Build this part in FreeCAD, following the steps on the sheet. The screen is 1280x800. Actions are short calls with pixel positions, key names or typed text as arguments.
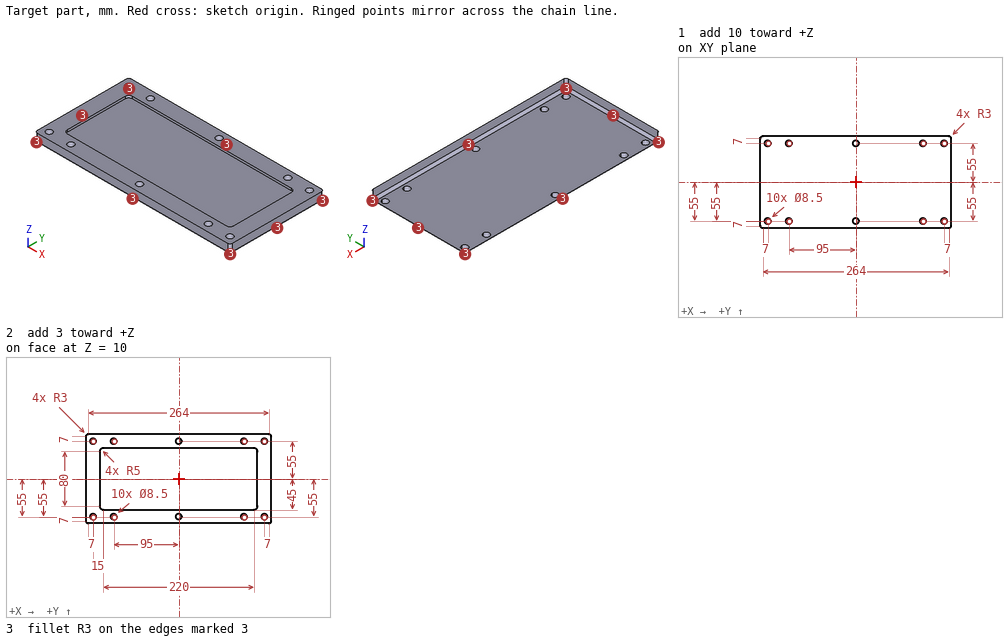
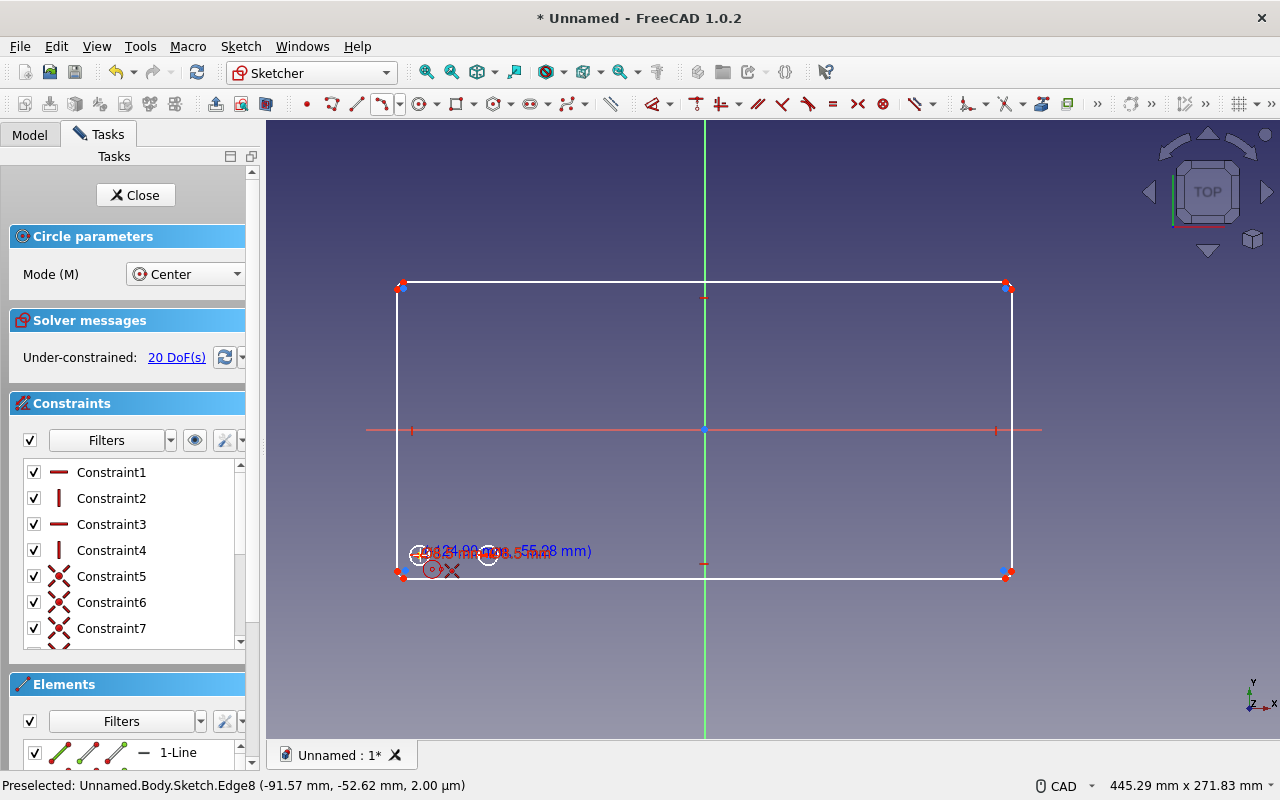
scroll(705, 555, up, 5)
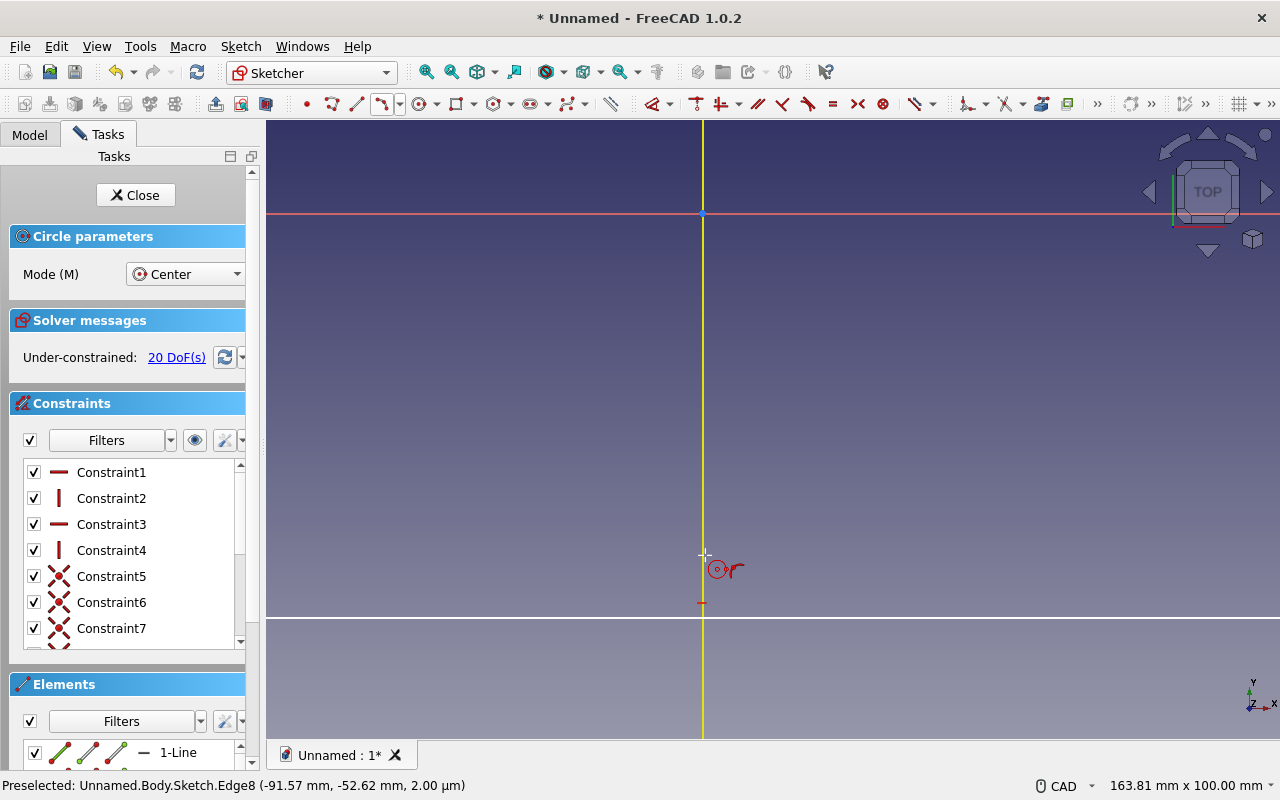
click(703, 554)
move(722, 536)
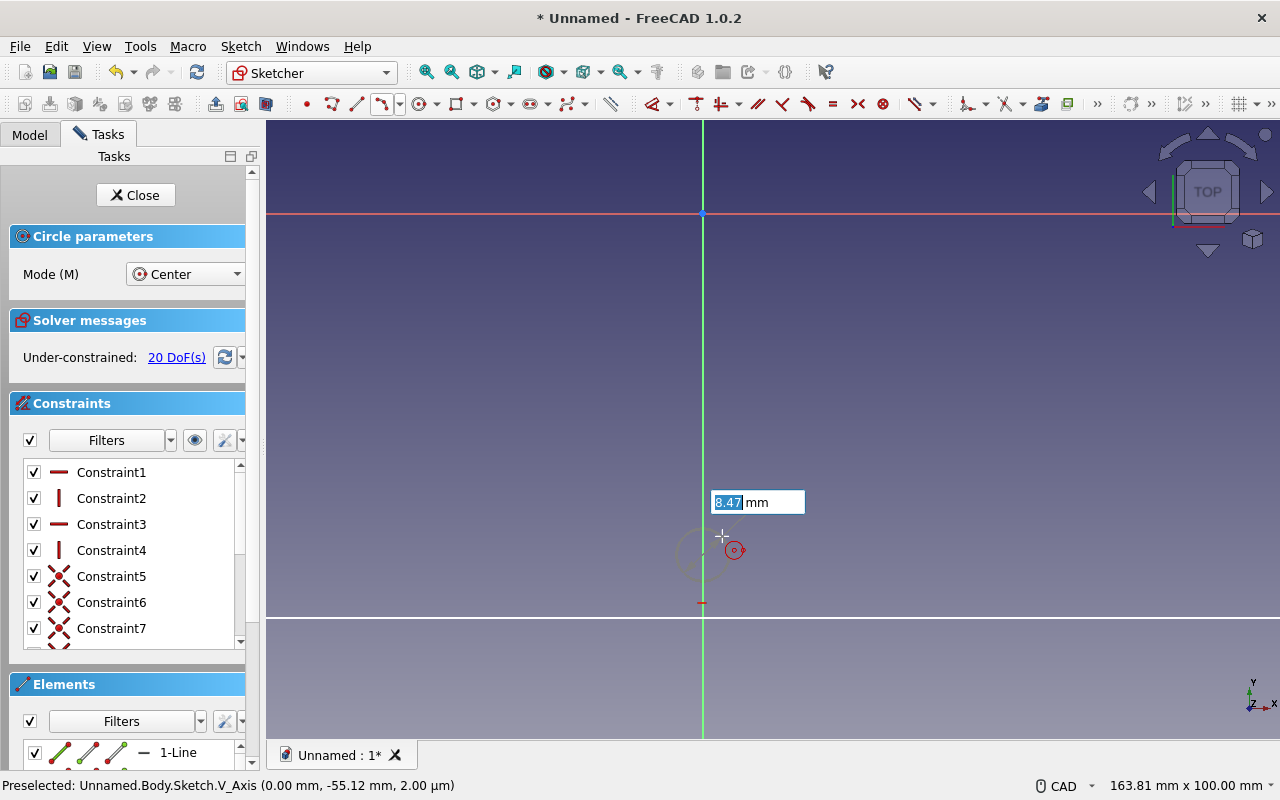
text(8.5)
key(Return)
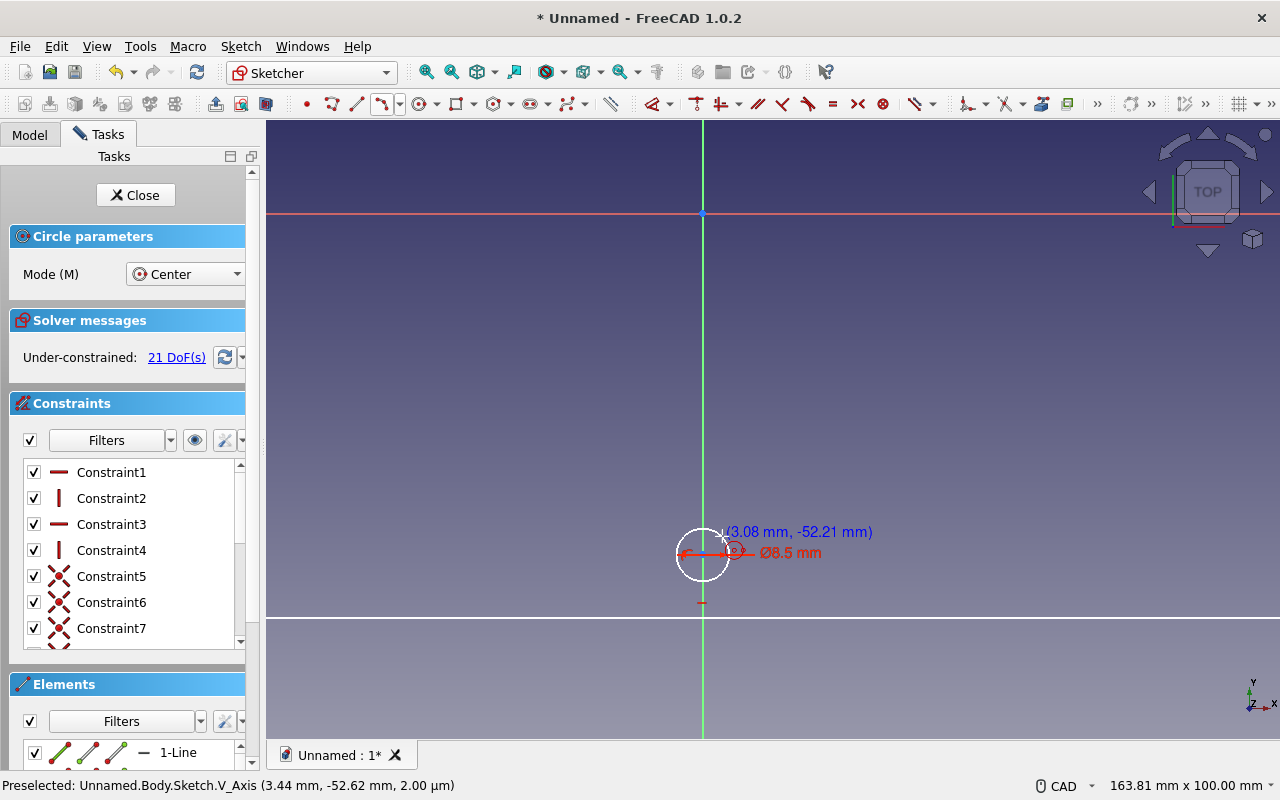
scroll(705, 555, down, 5)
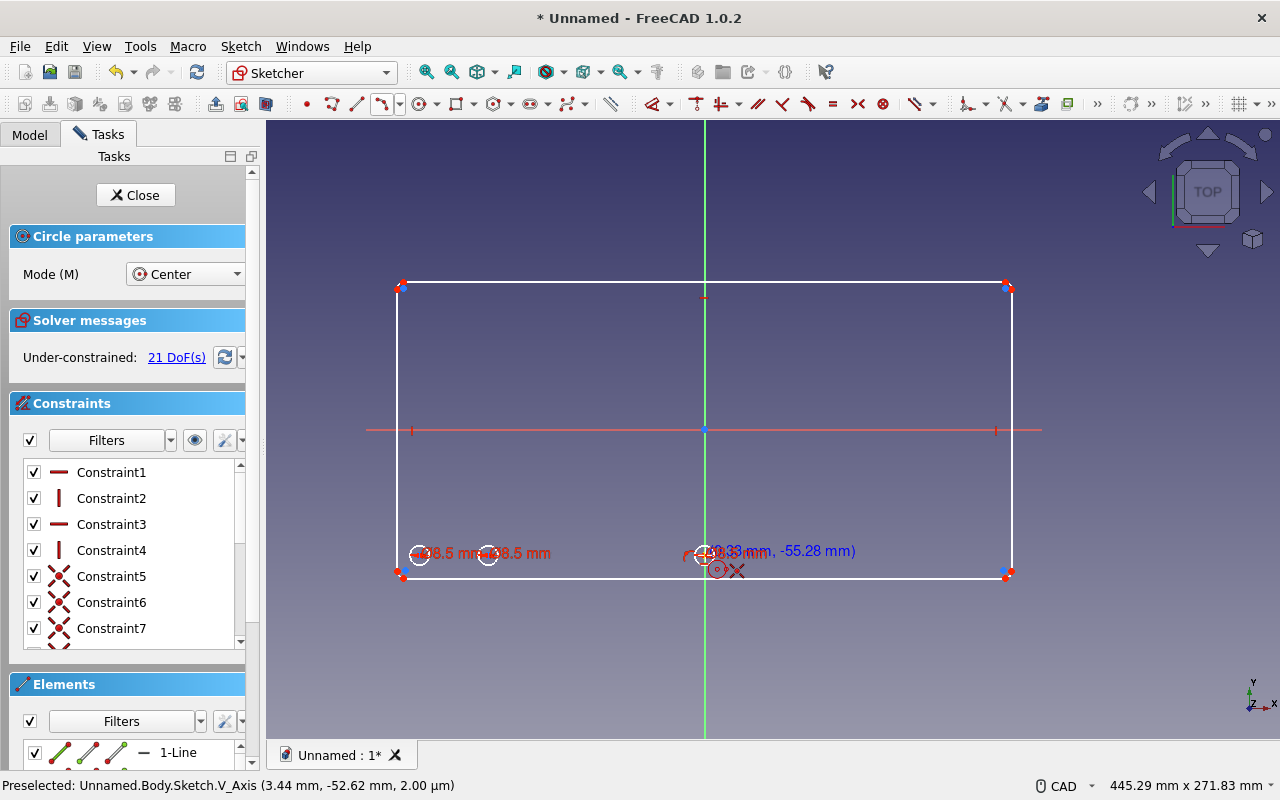
scroll(921, 555, up, 5)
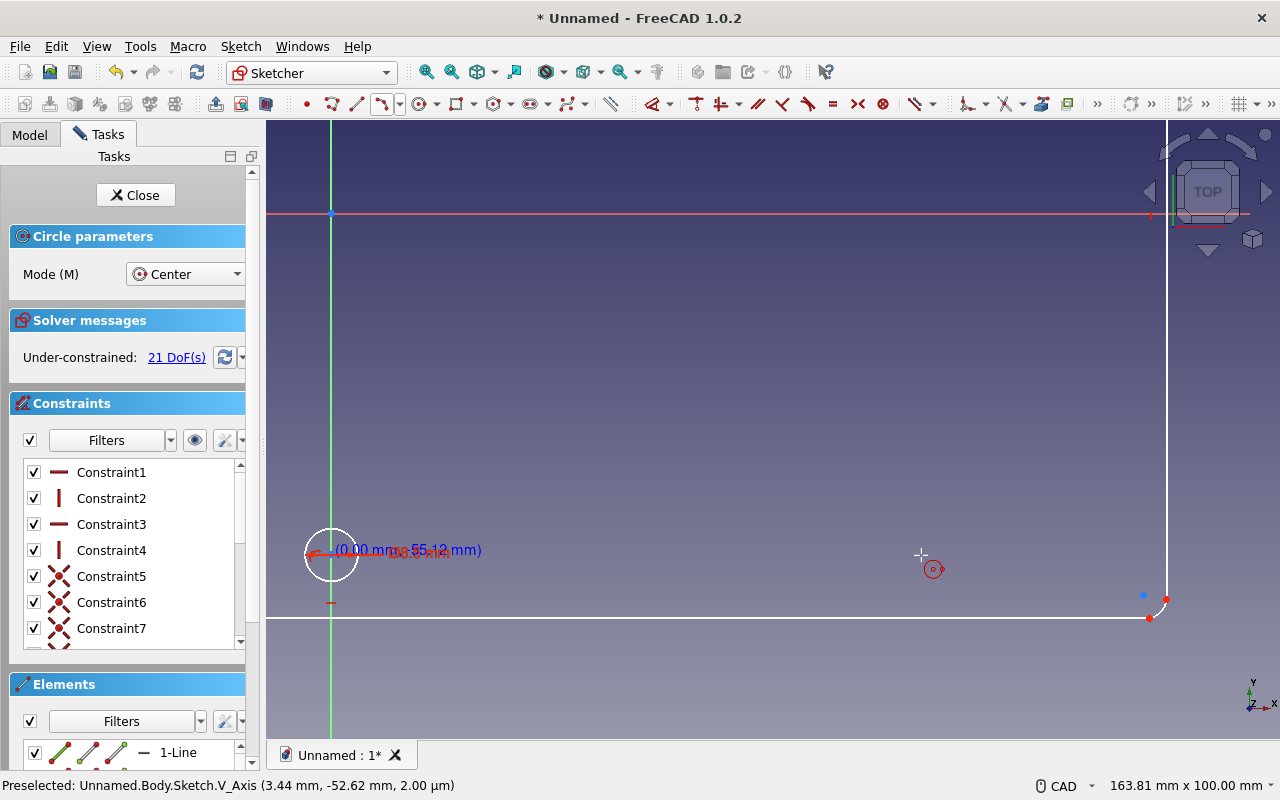
click(919, 554)
move(938, 536)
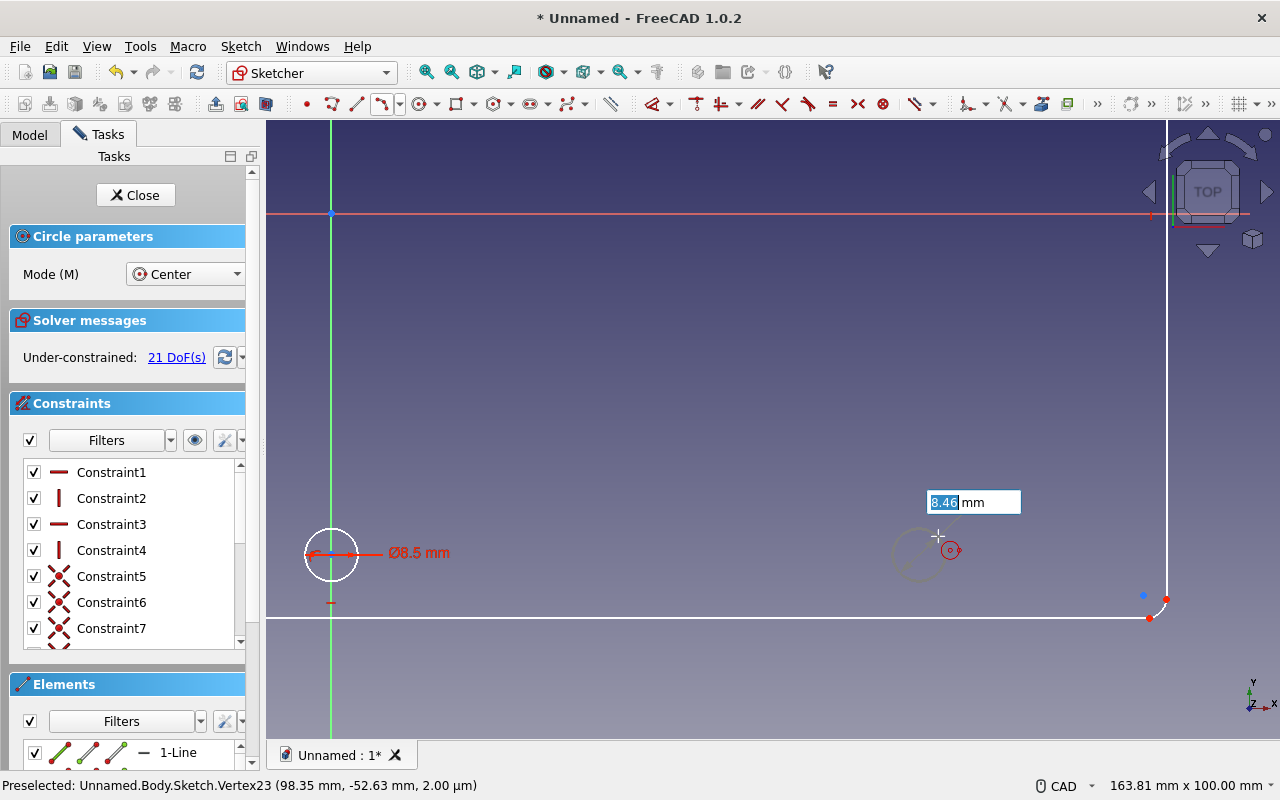
text(8.5)
key(Return)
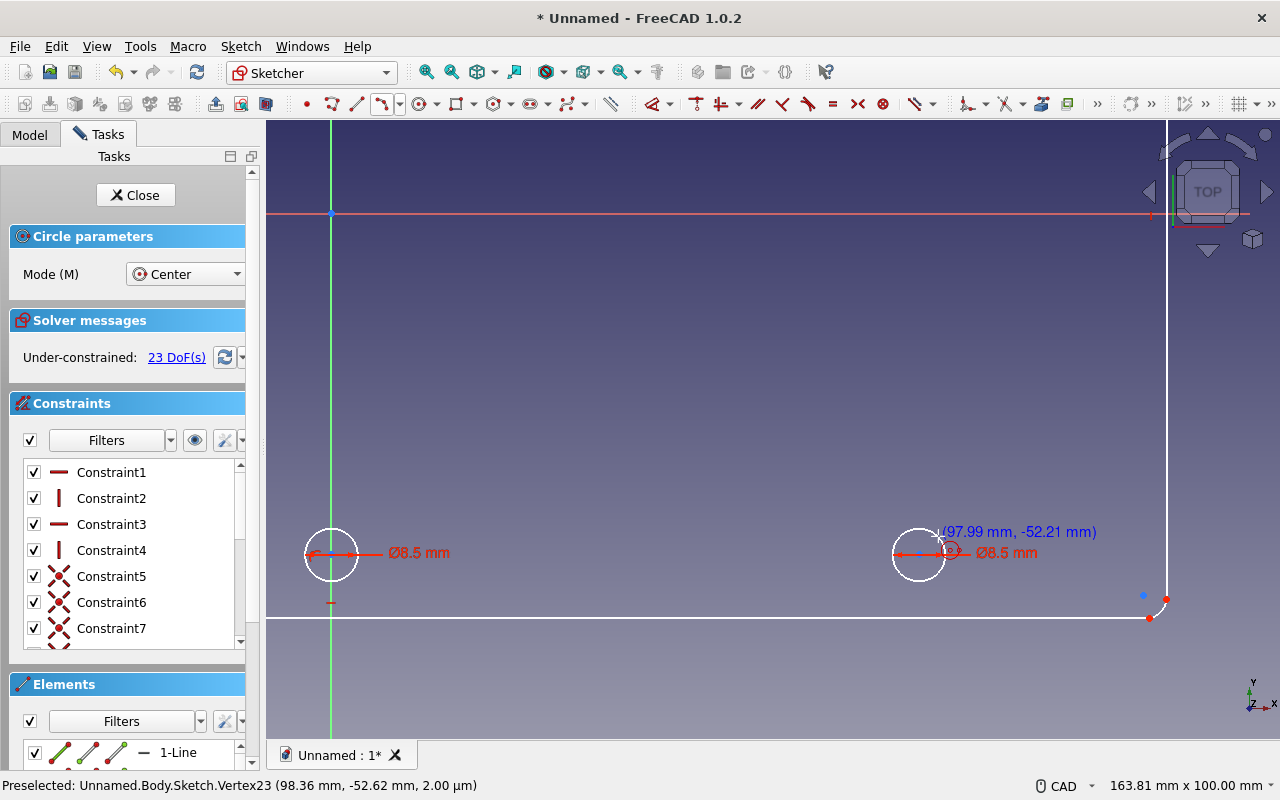
click(1105, 554)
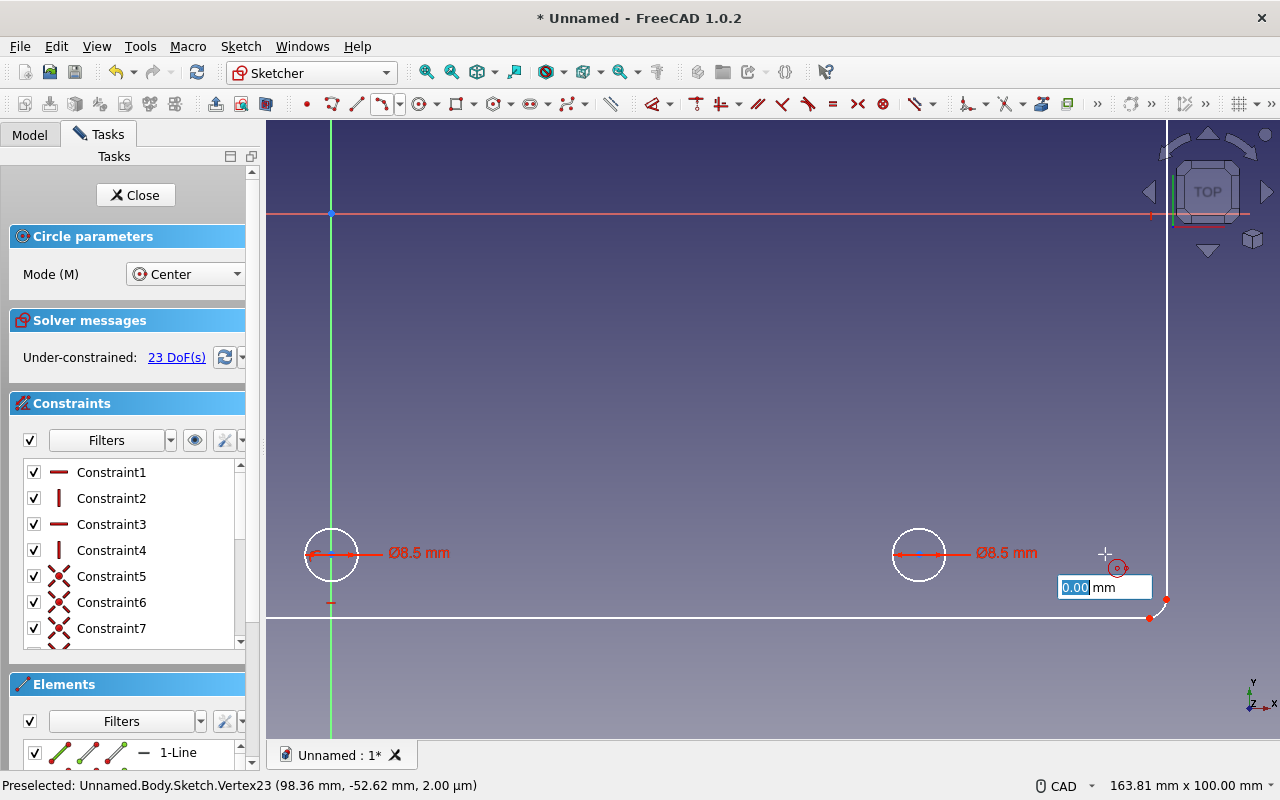
scroll(922, 555, down, 5)
move(997, 548)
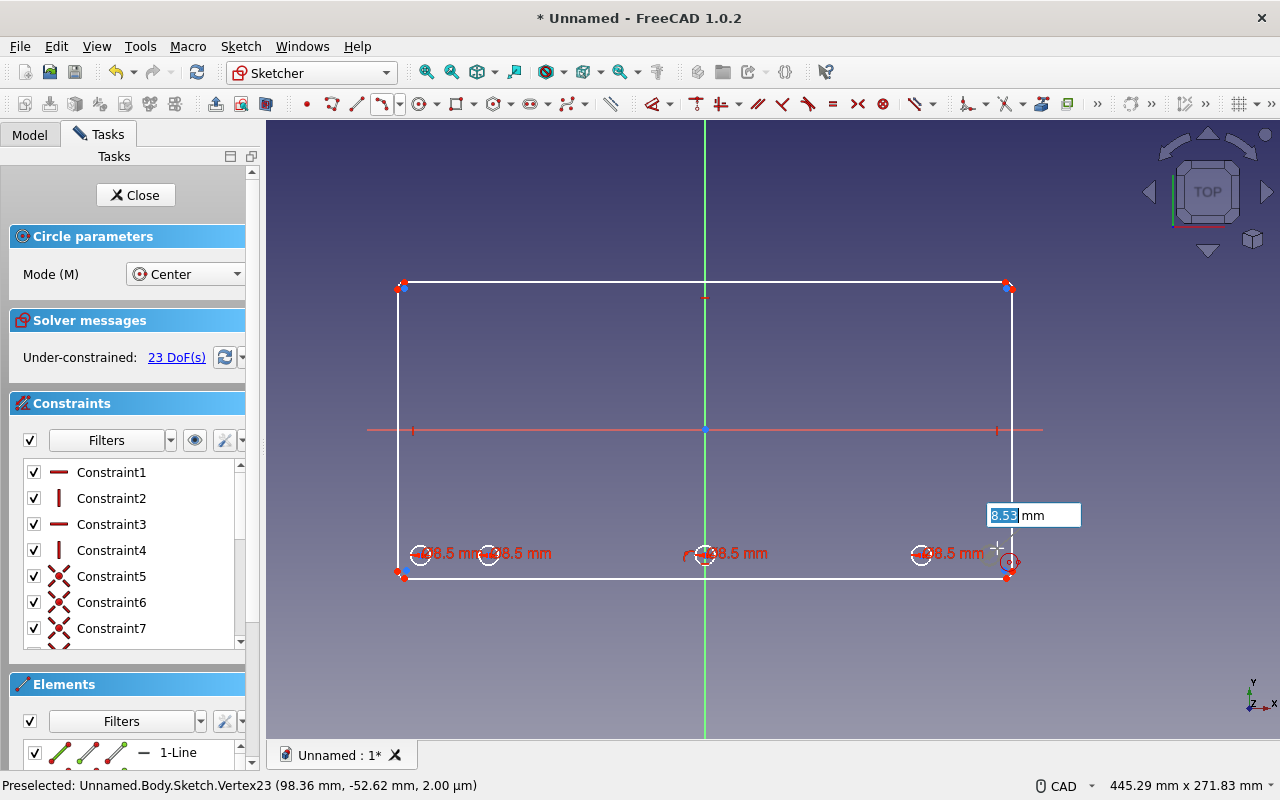
text(8.5)
key(Return)